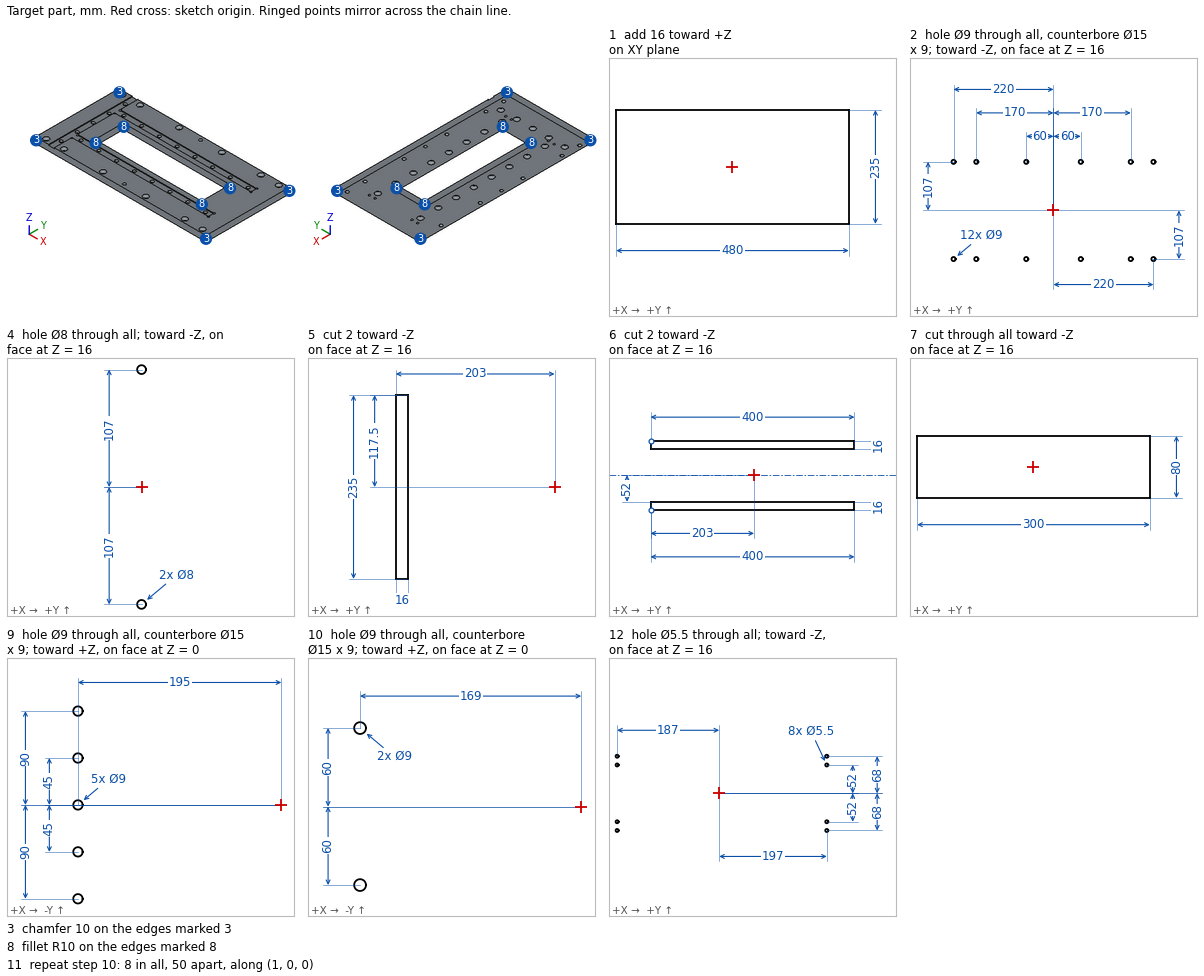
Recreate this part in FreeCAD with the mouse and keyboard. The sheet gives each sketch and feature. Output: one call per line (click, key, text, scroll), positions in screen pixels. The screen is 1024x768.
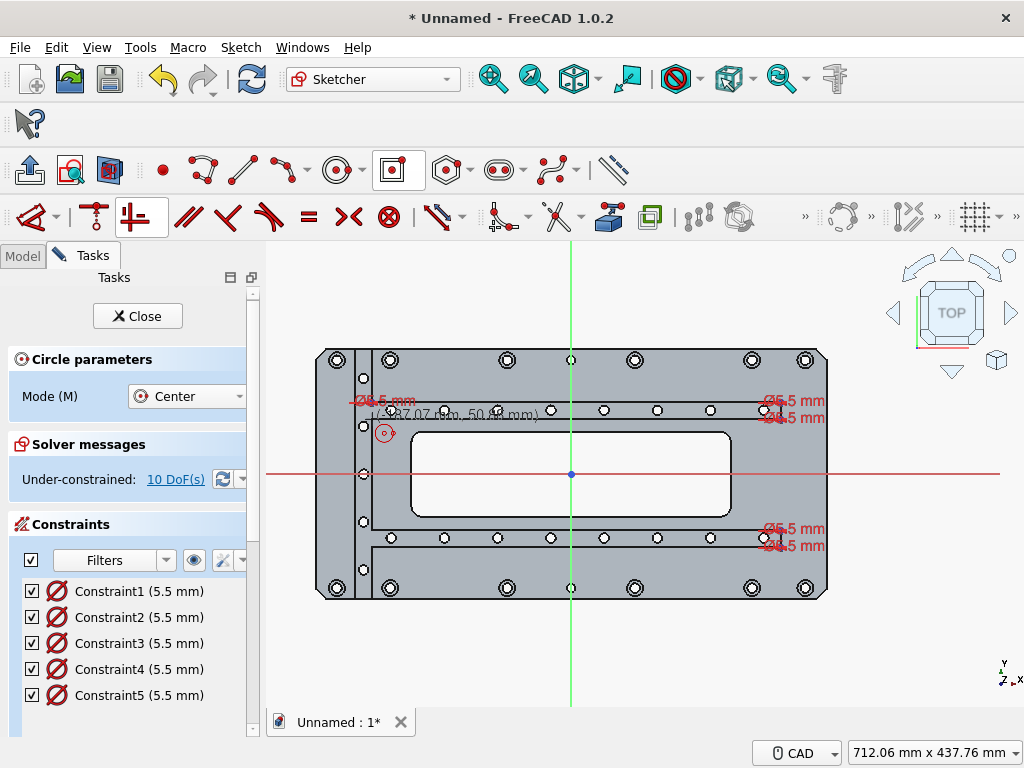
click(372, 419)
move(374, 421)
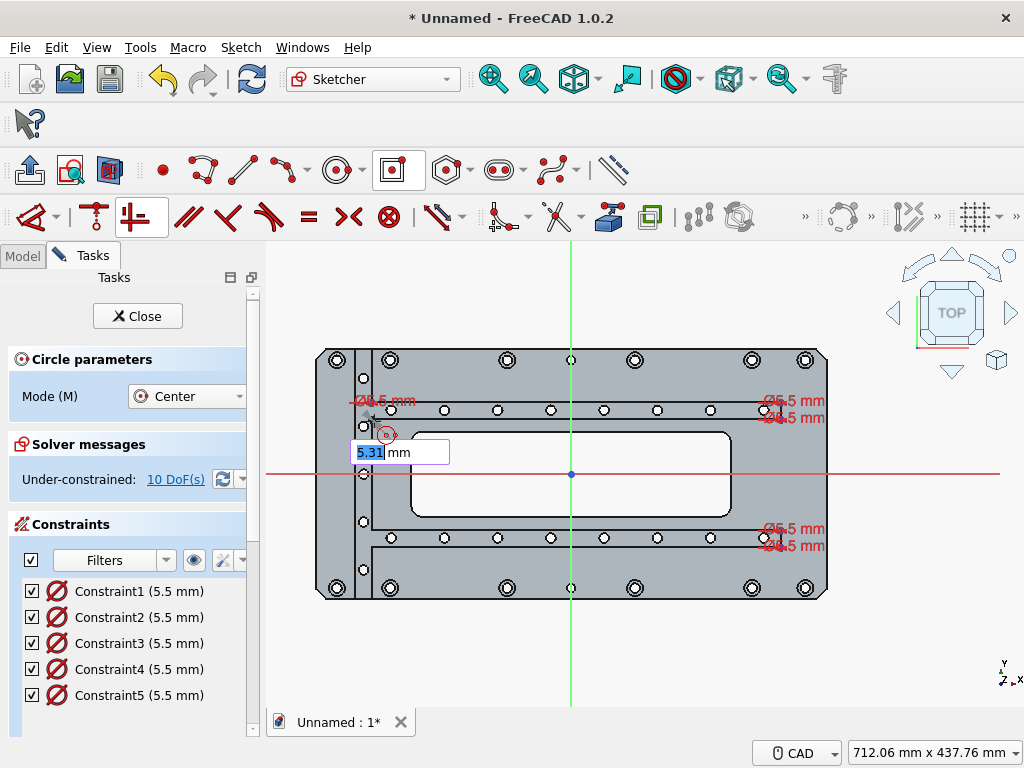
text(5.5)
key(Return)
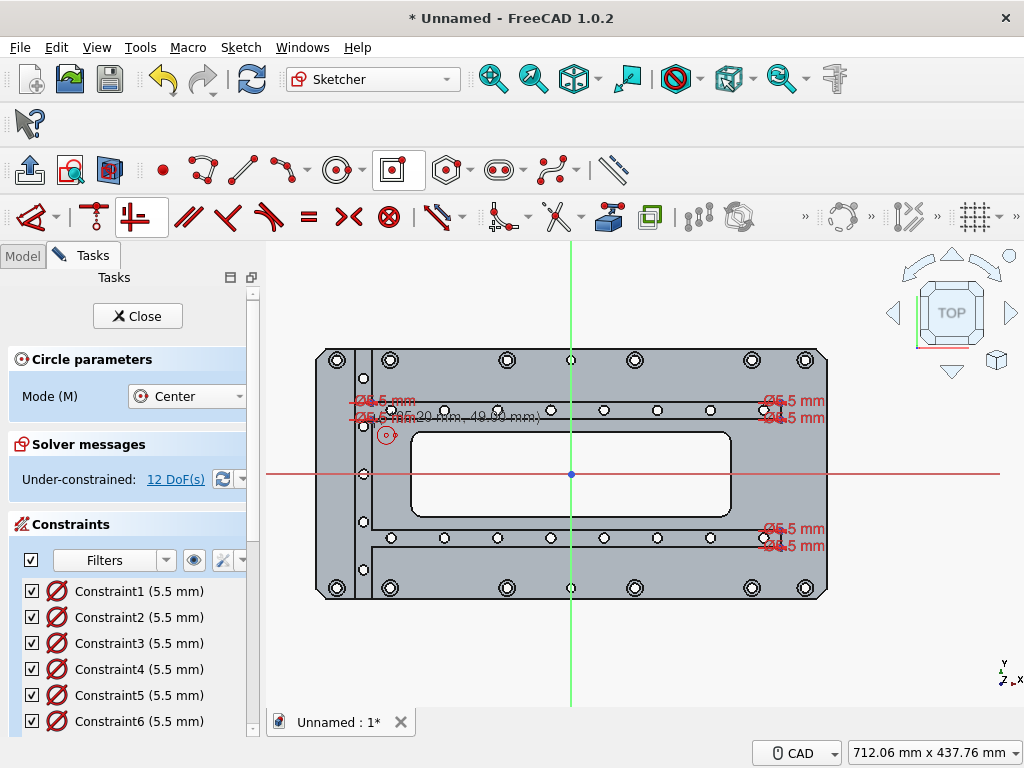
scroll(372, 547, up, 11)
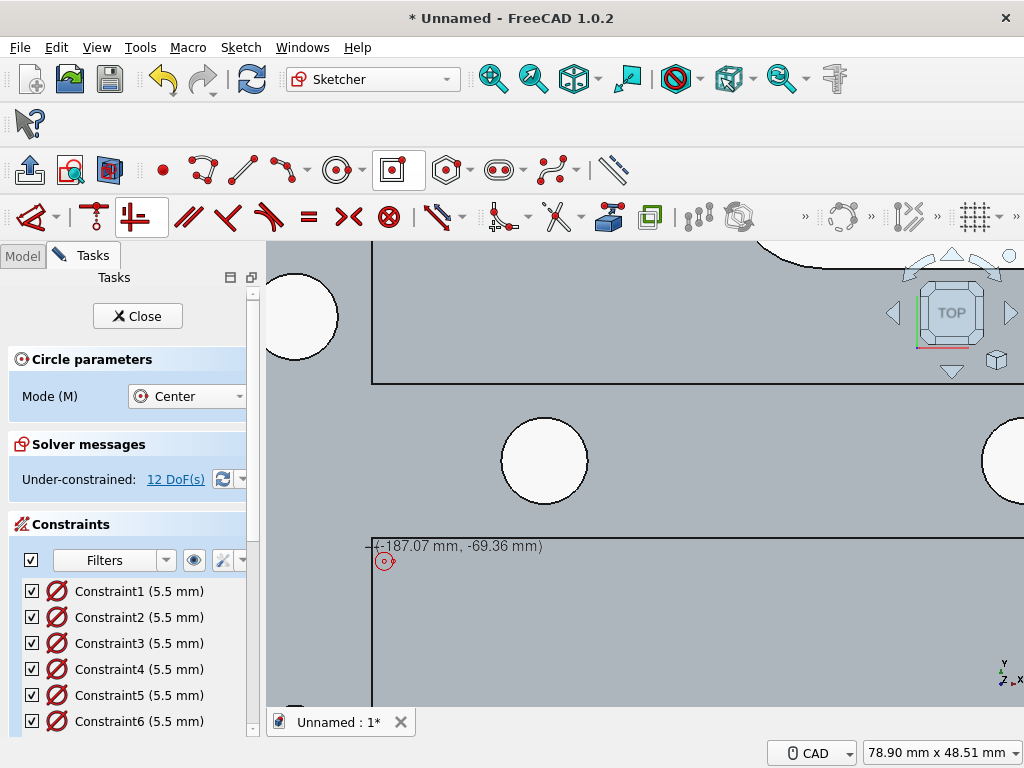
scroll(372, 547, down, 11)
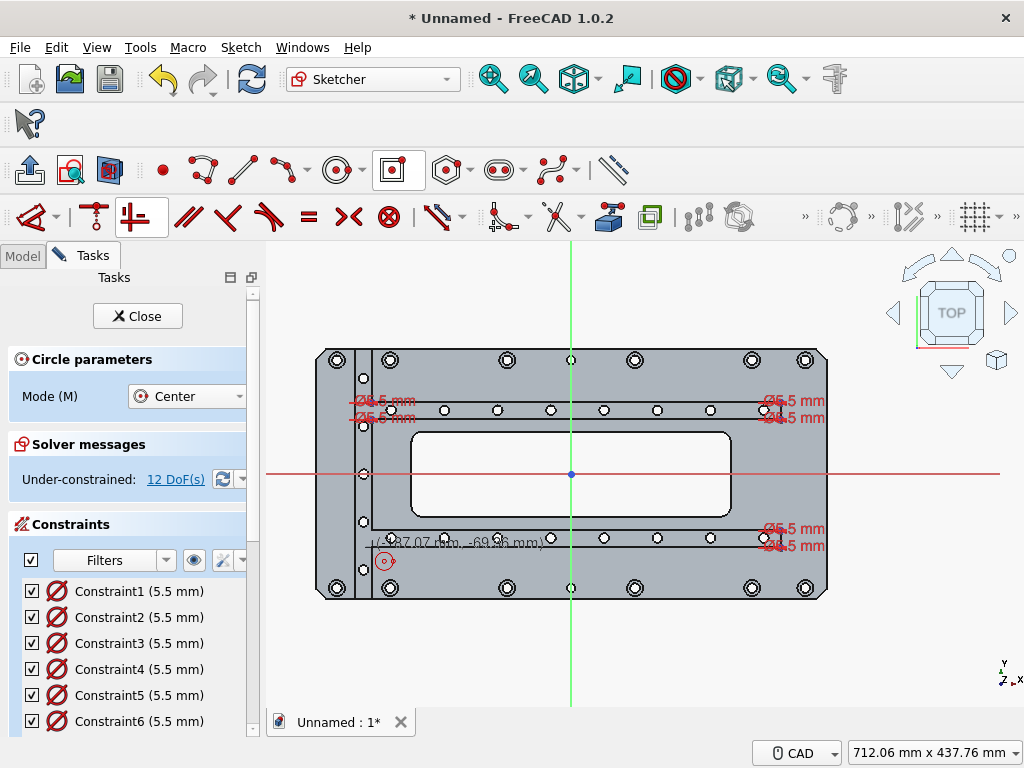
click(372, 547)
move(374, 544)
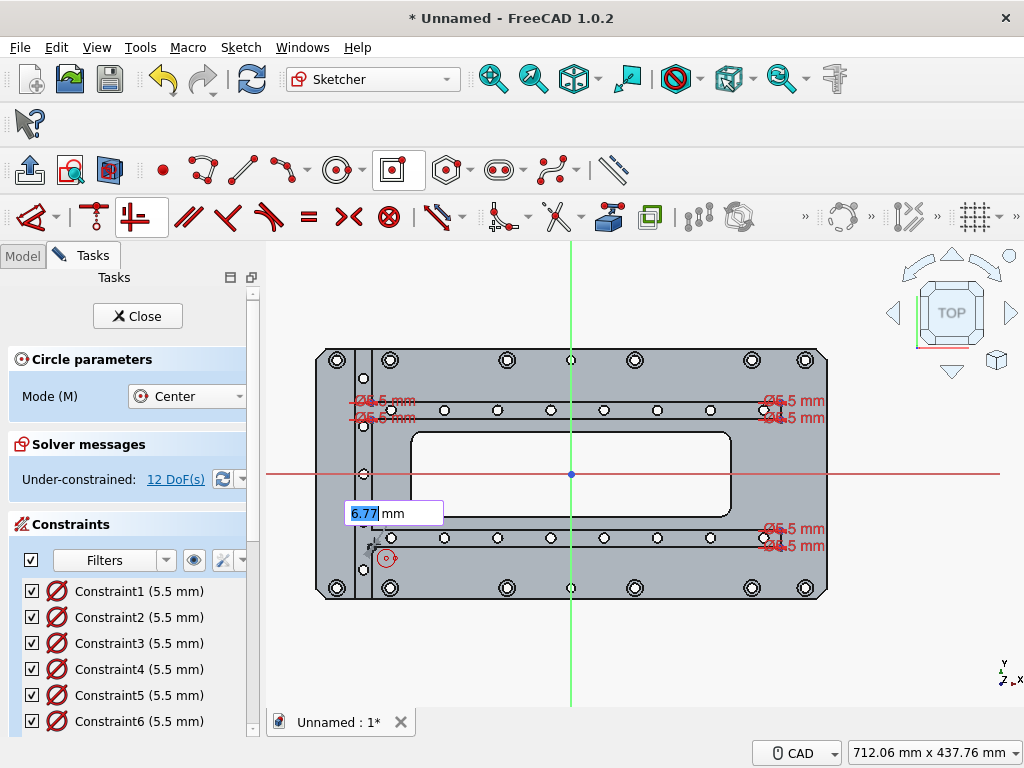
text(5.5)
key(Return)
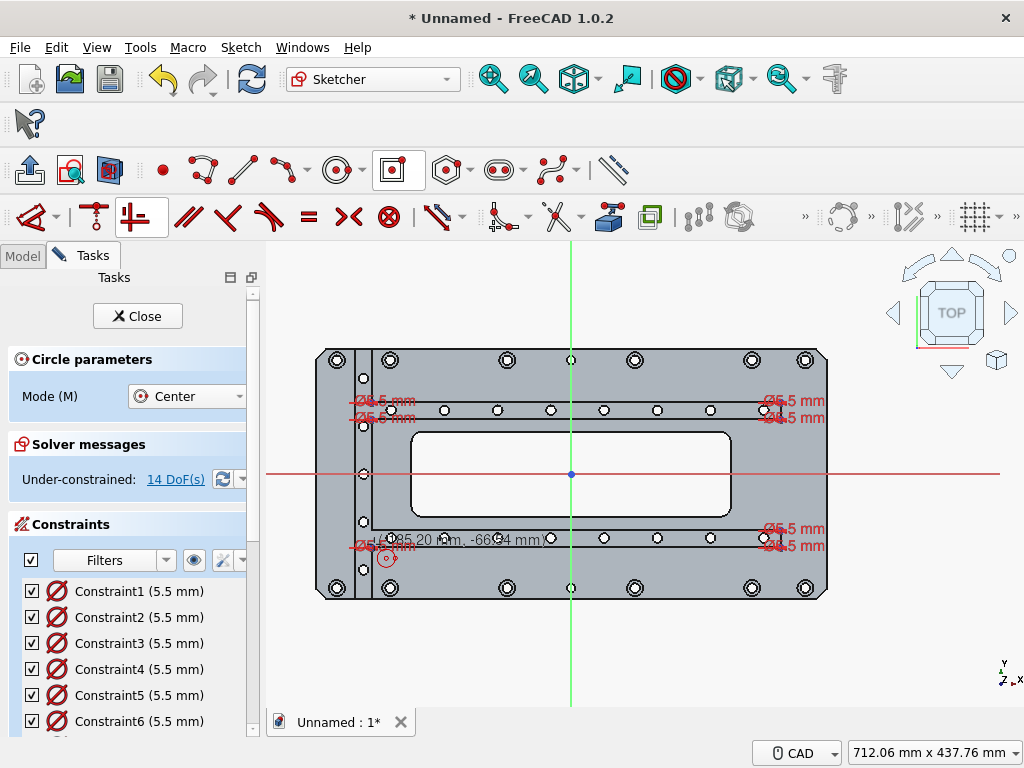
scroll(372, 530, up, 11)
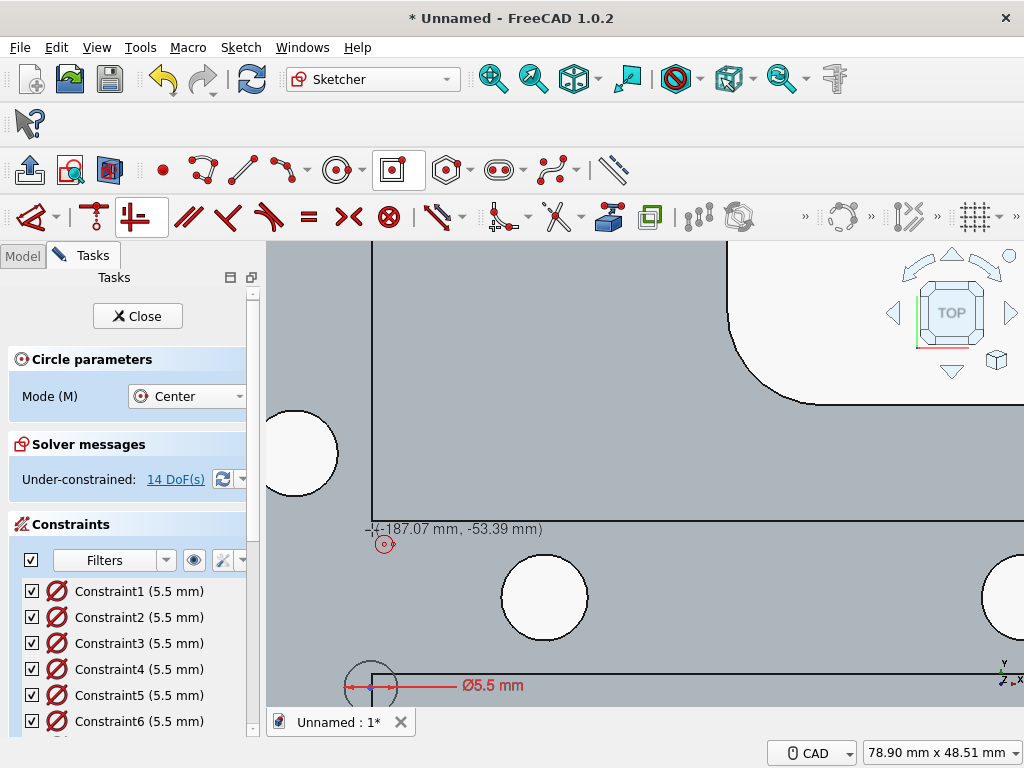
scroll(372, 530, down, 11)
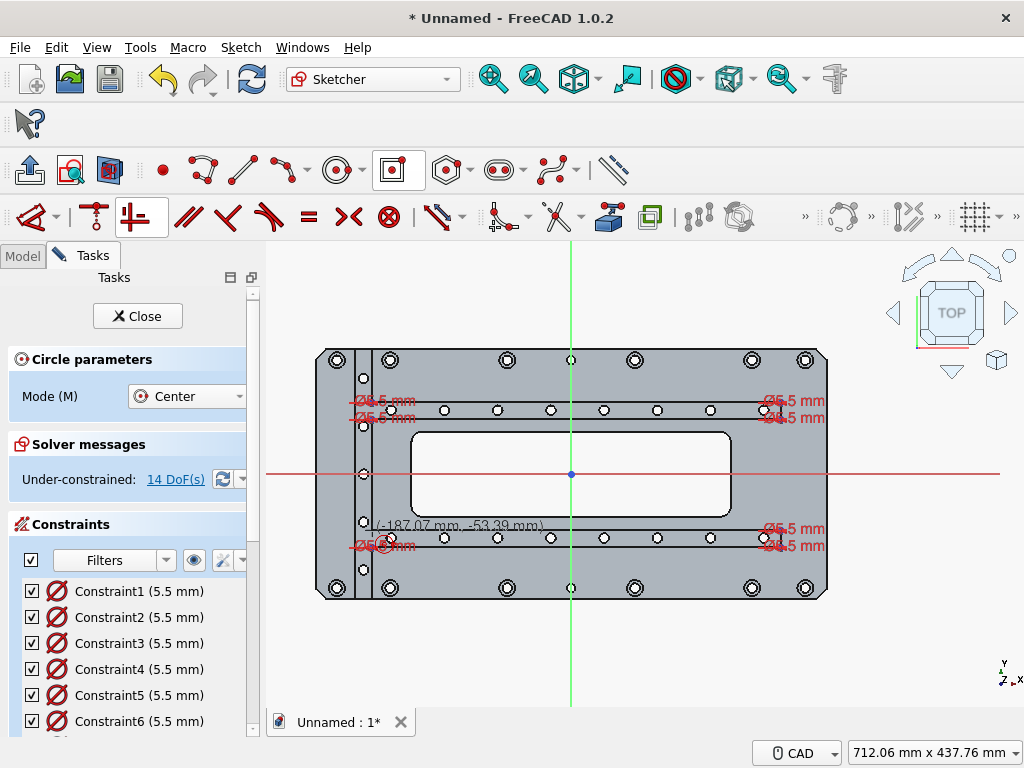
click(372, 530)
move(374, 527)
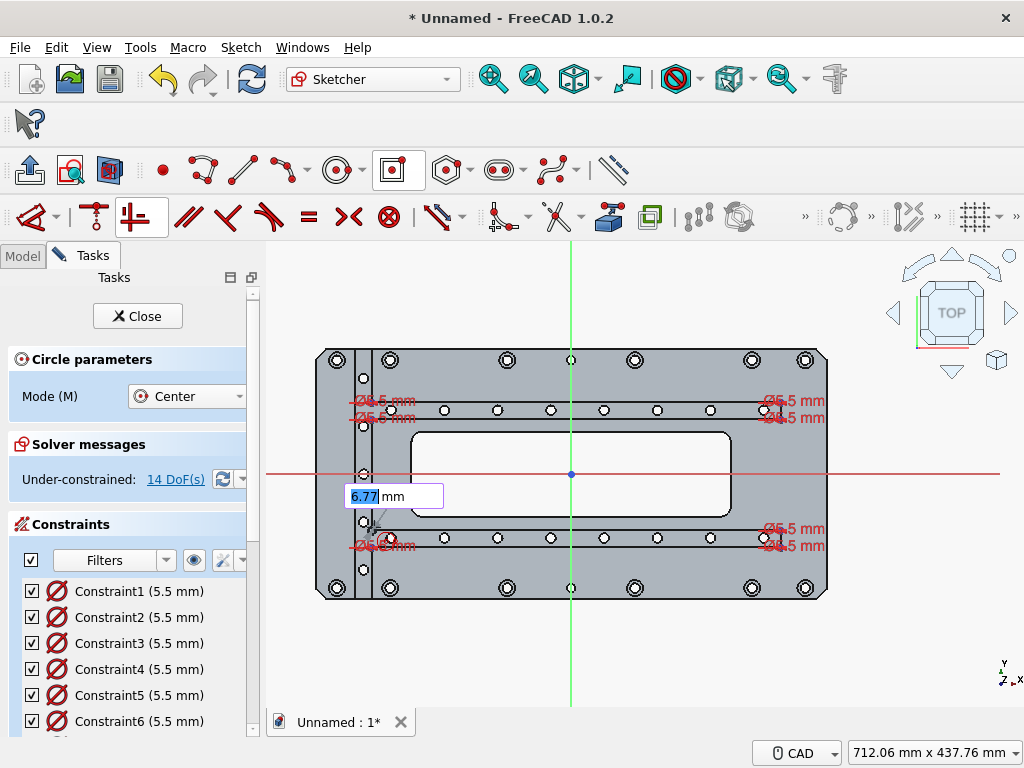
text(5.5)
key(Return)
key(Escape)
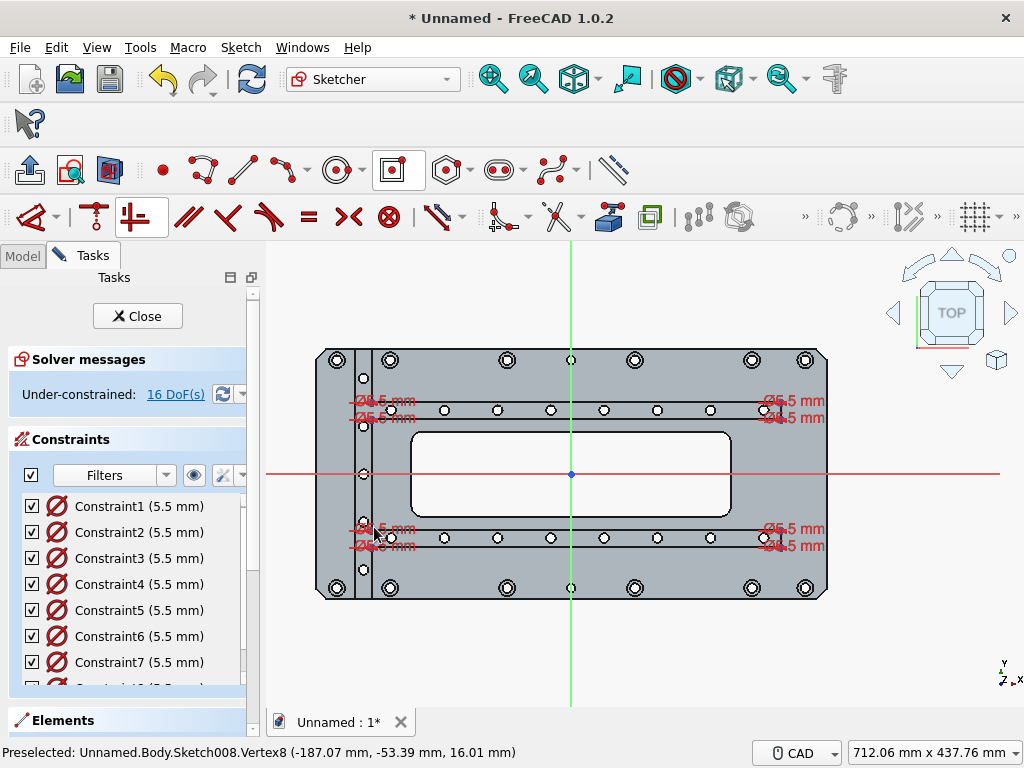
click(781, 548)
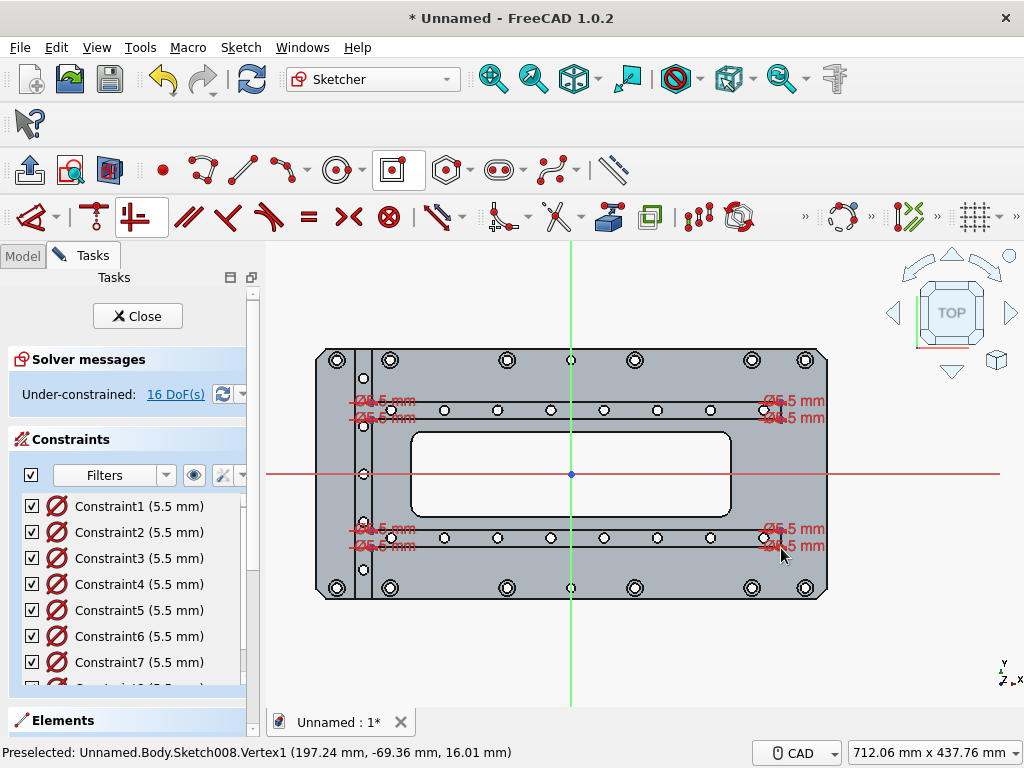
click(781, 531)